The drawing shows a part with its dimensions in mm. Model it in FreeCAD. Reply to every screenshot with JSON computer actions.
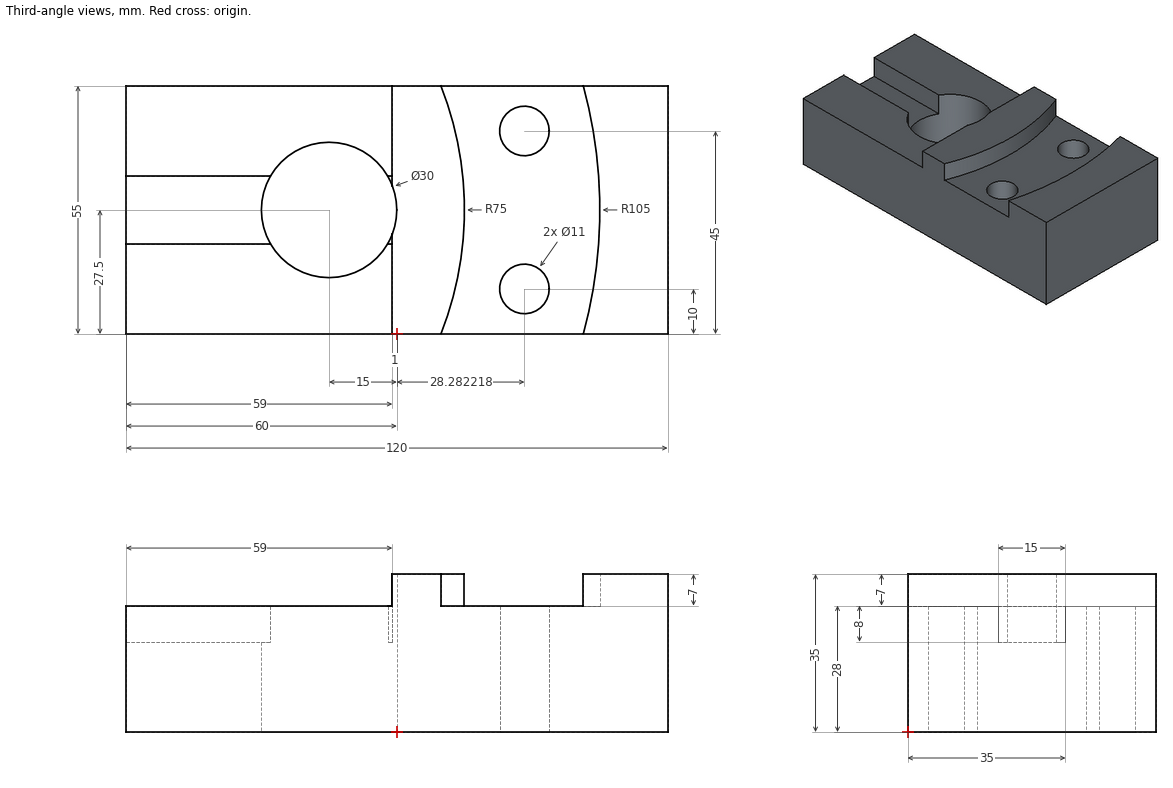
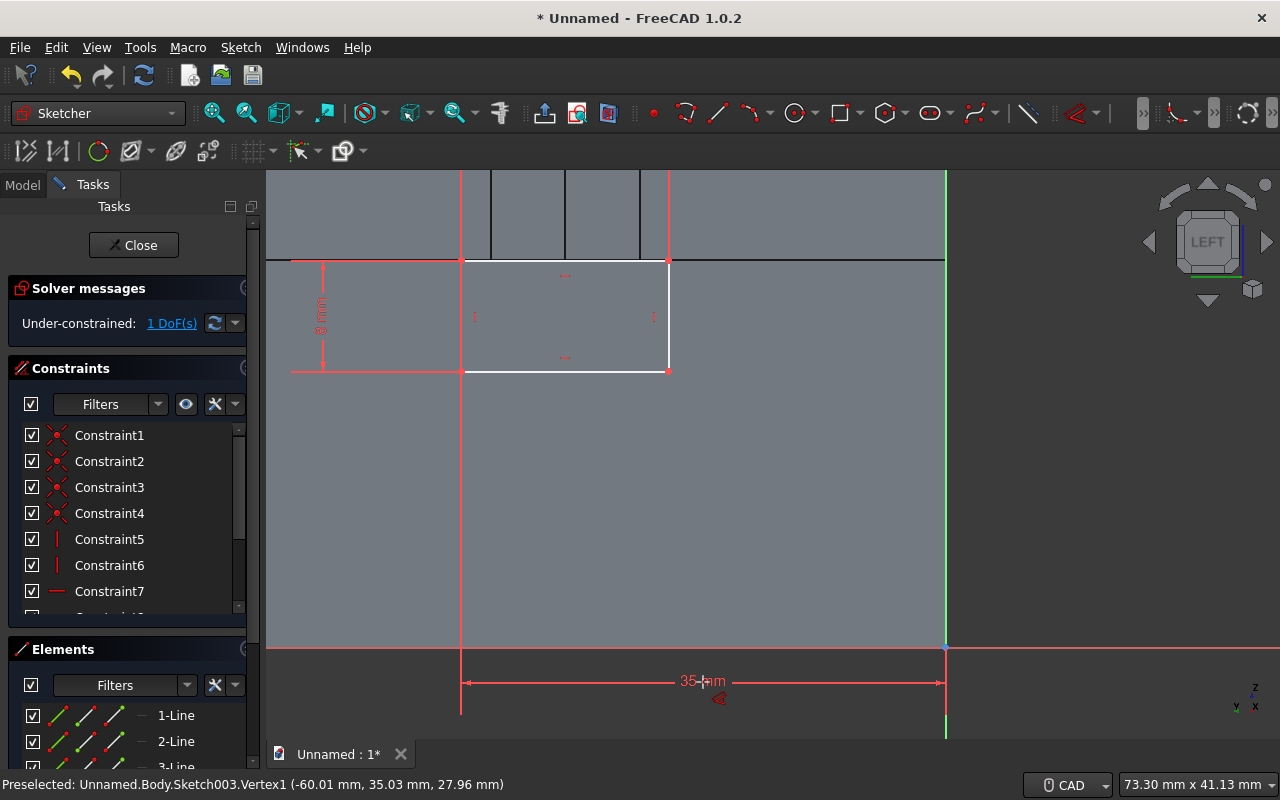
{"action": "left_click", "coordinate": [461, 261]}
{"action": "left_click", "coordinate": [980, 454]}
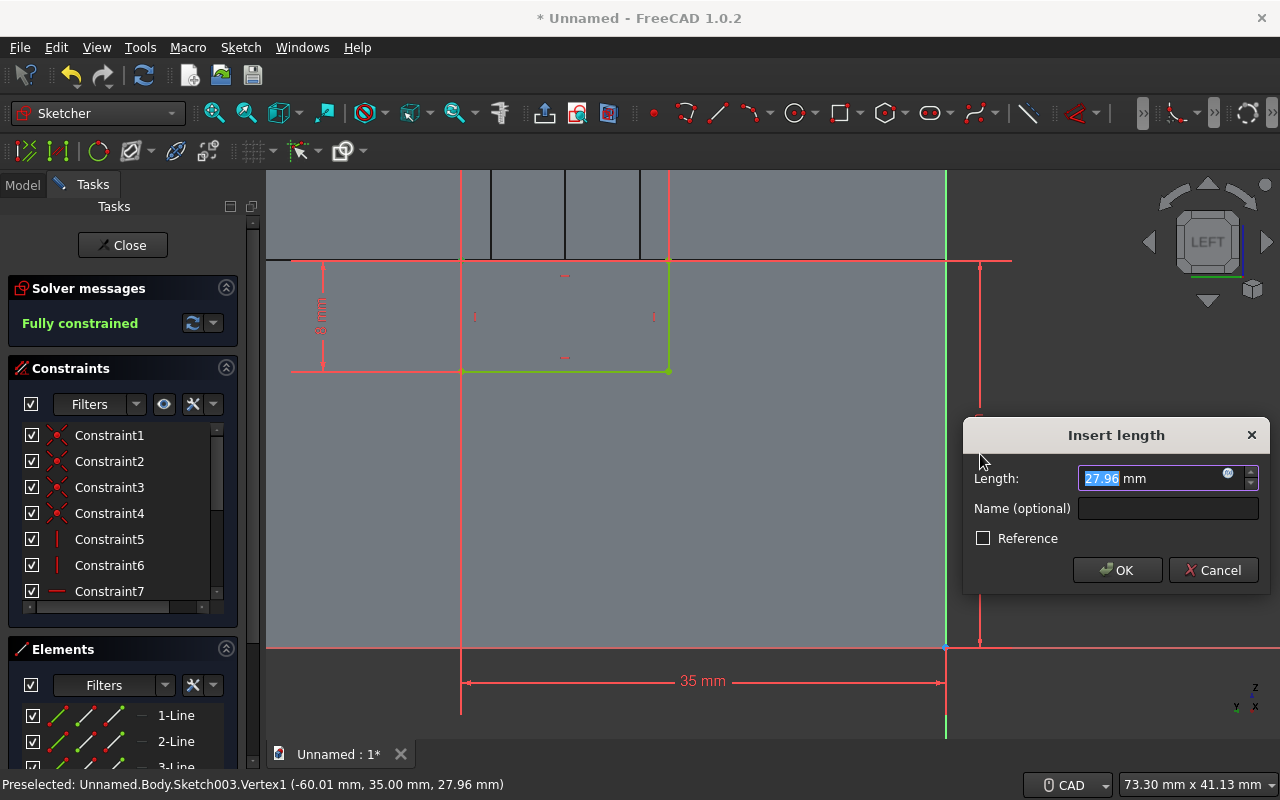
{"action": "type", "text": "28"}
{"action": "key", "text": "Return"}
{"action": "key", "text": "Escape"}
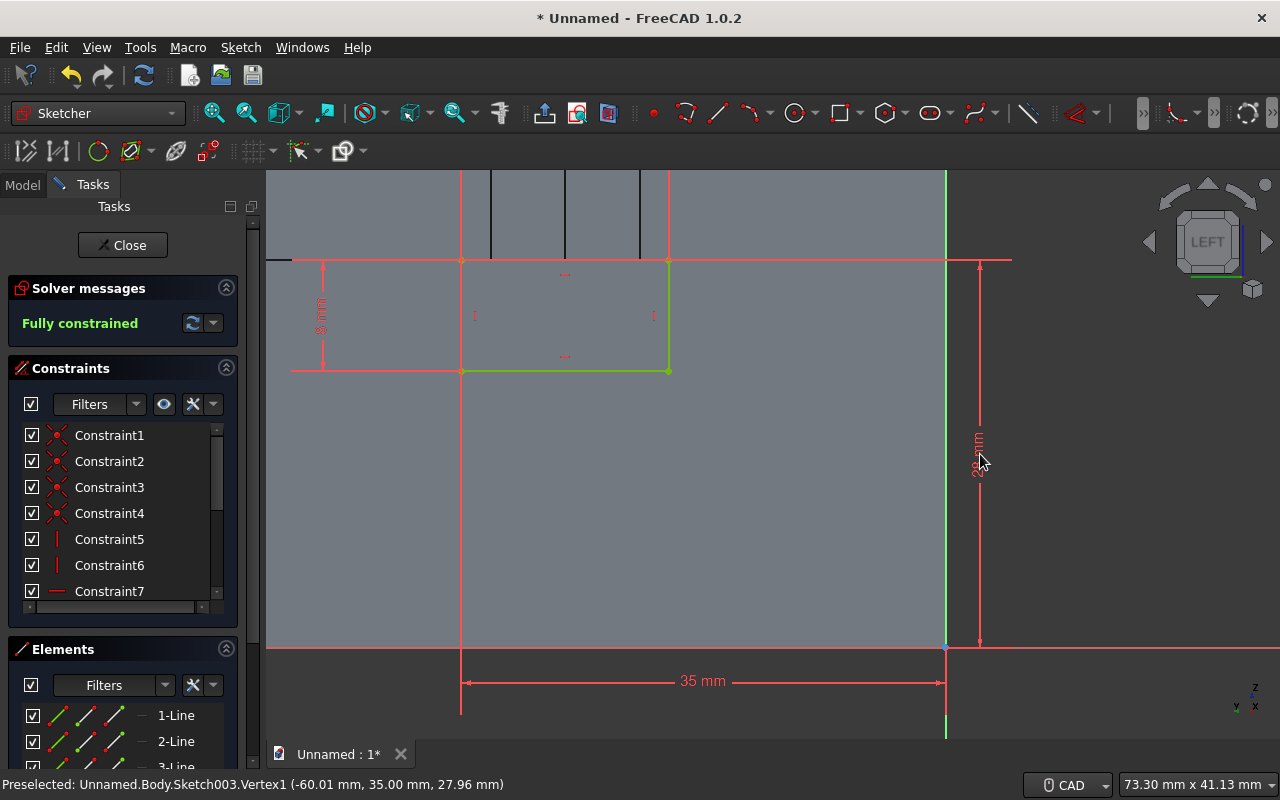
{"action": "left_click", "coordinate": [123, 245]}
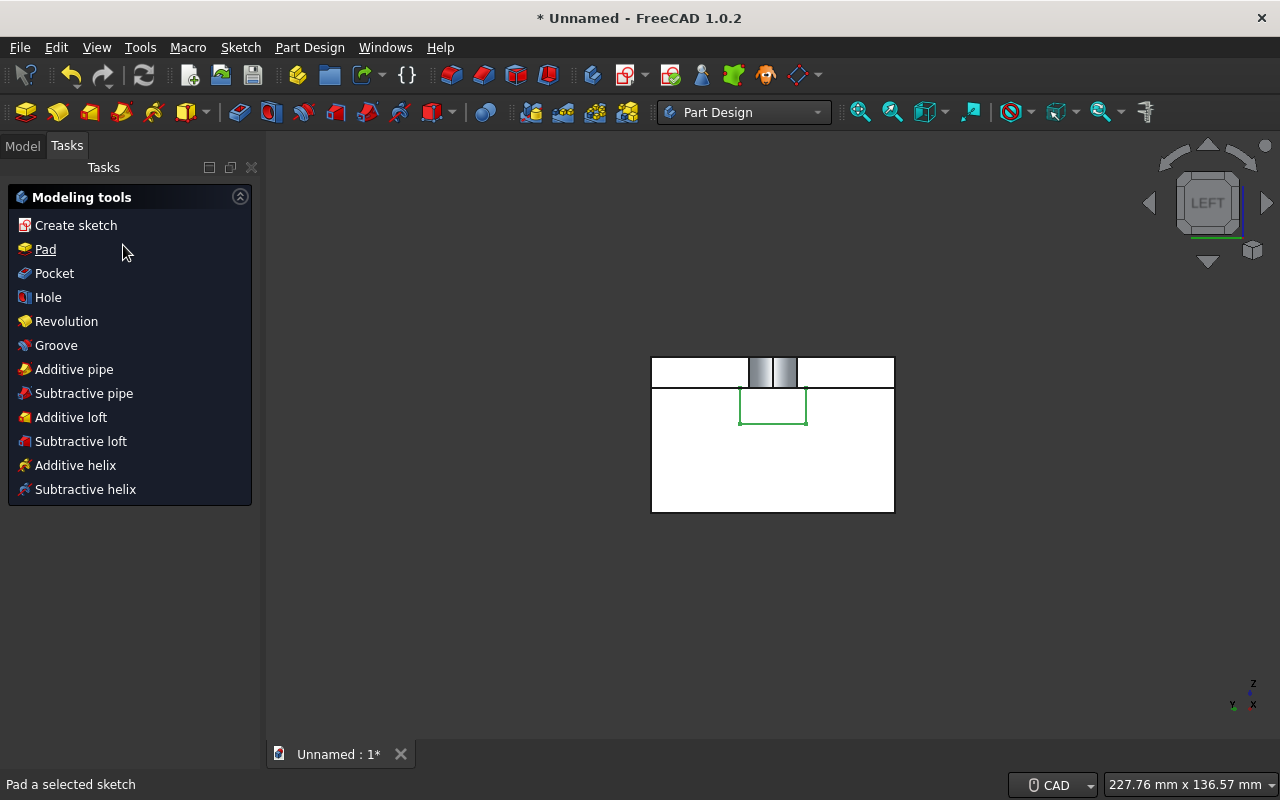
{"action": "left_click", "coordinate": [240, 112]}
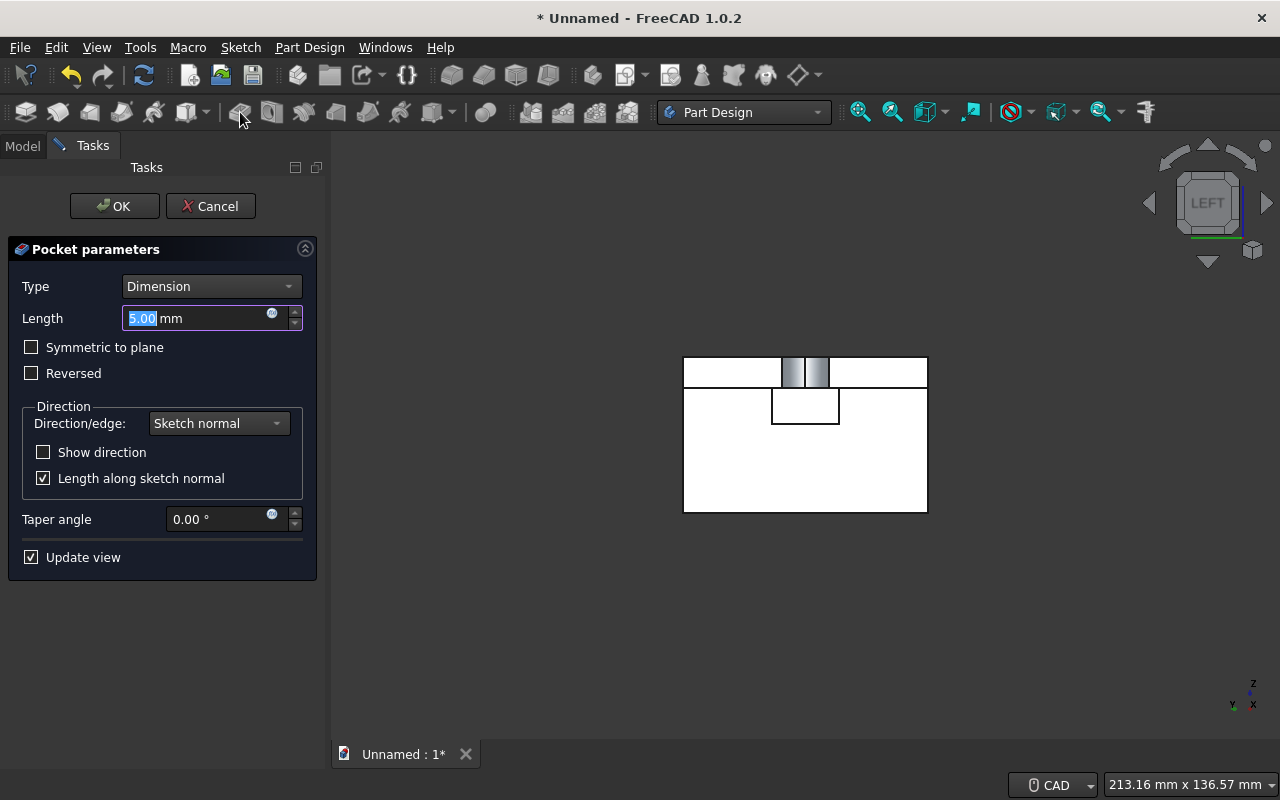
{"action": "type", "text": "59"}
{"action": "key", "text": "Tab"}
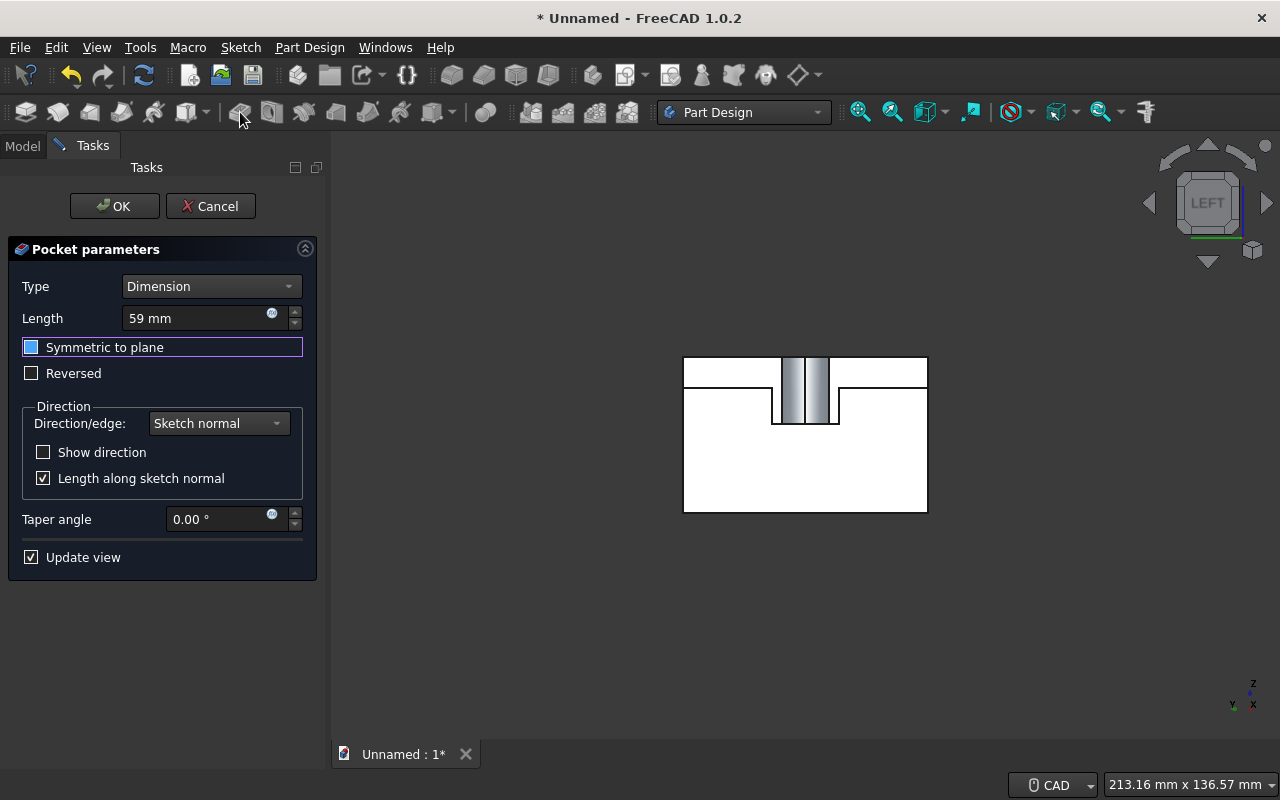
{"action": "left_click", "coordinate": [115, 206]}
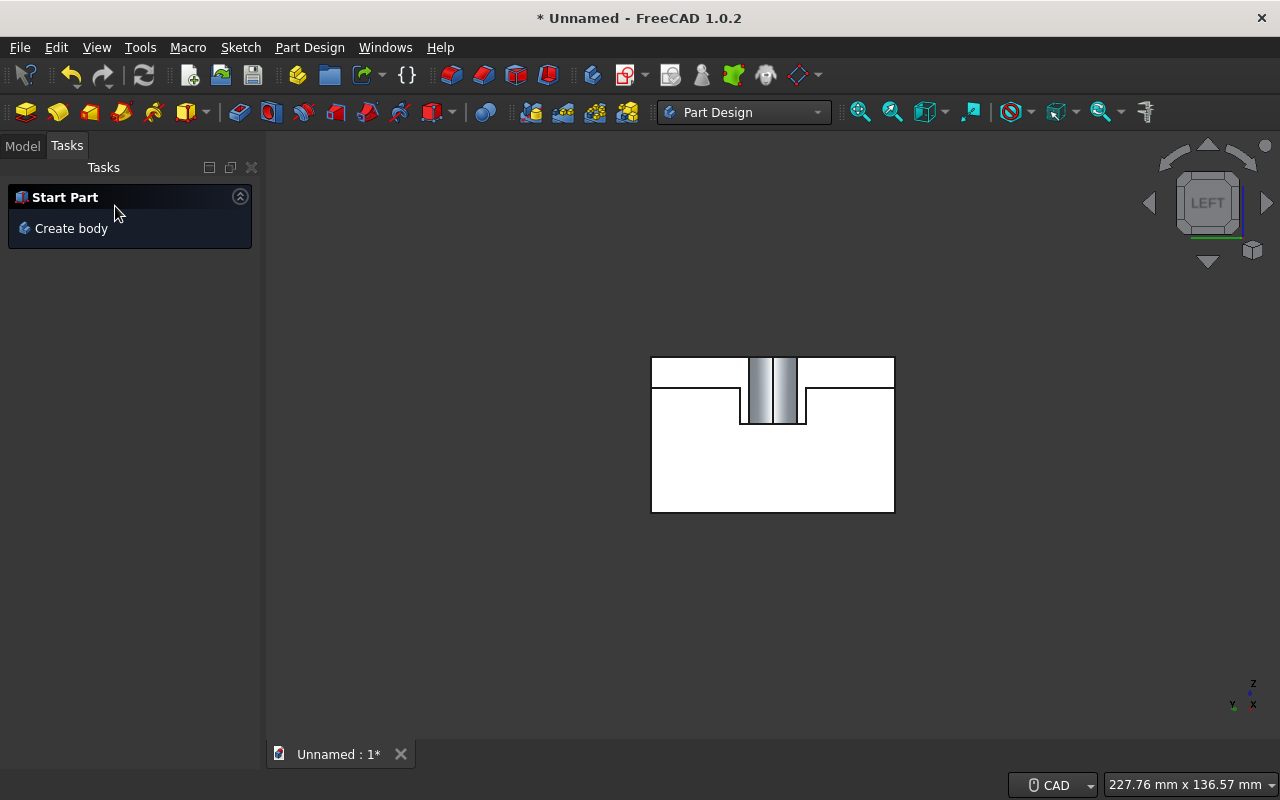
{"action": "key", "text": "0"}